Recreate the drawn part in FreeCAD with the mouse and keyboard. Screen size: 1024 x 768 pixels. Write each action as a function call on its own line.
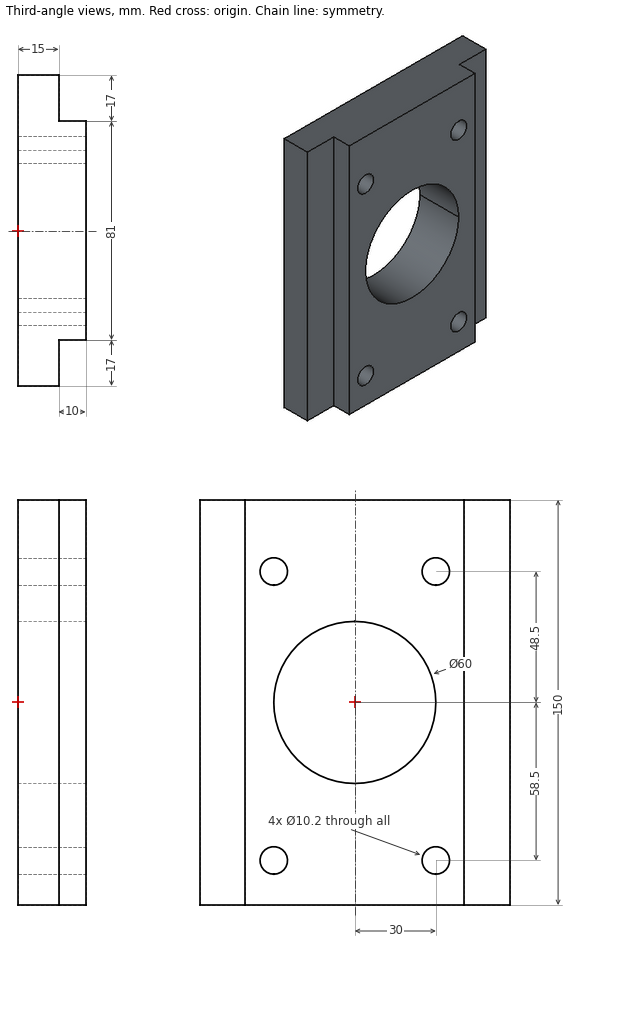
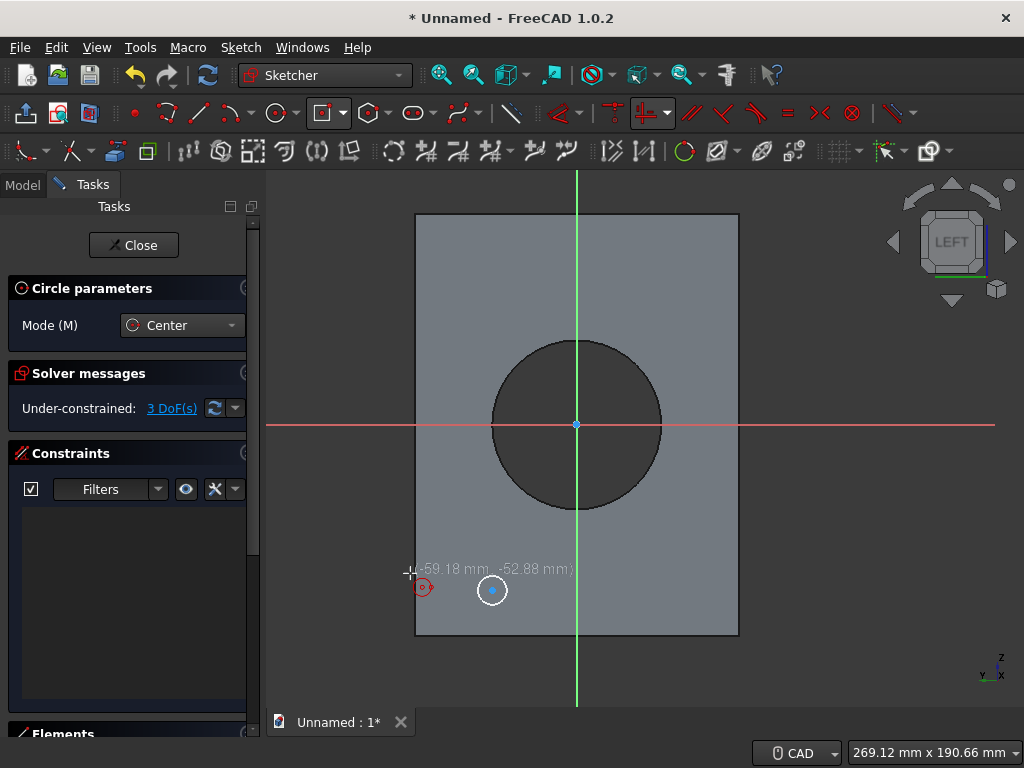
scroll(492, 288, up, 3)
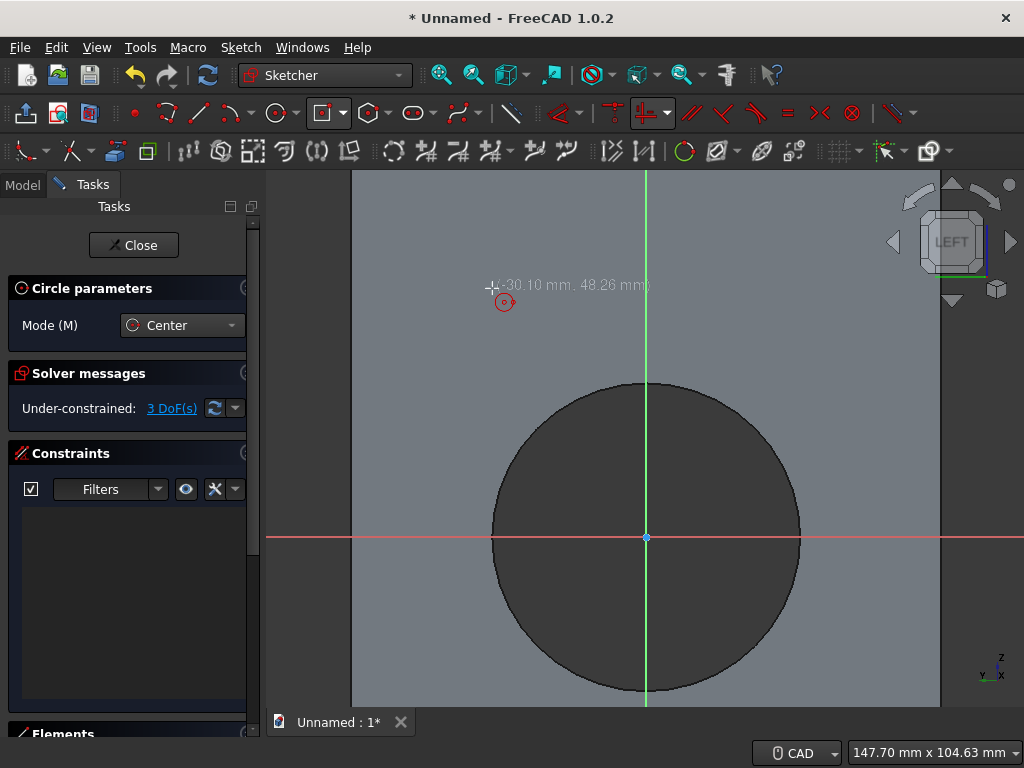
click(492, 288)
click(511, 270)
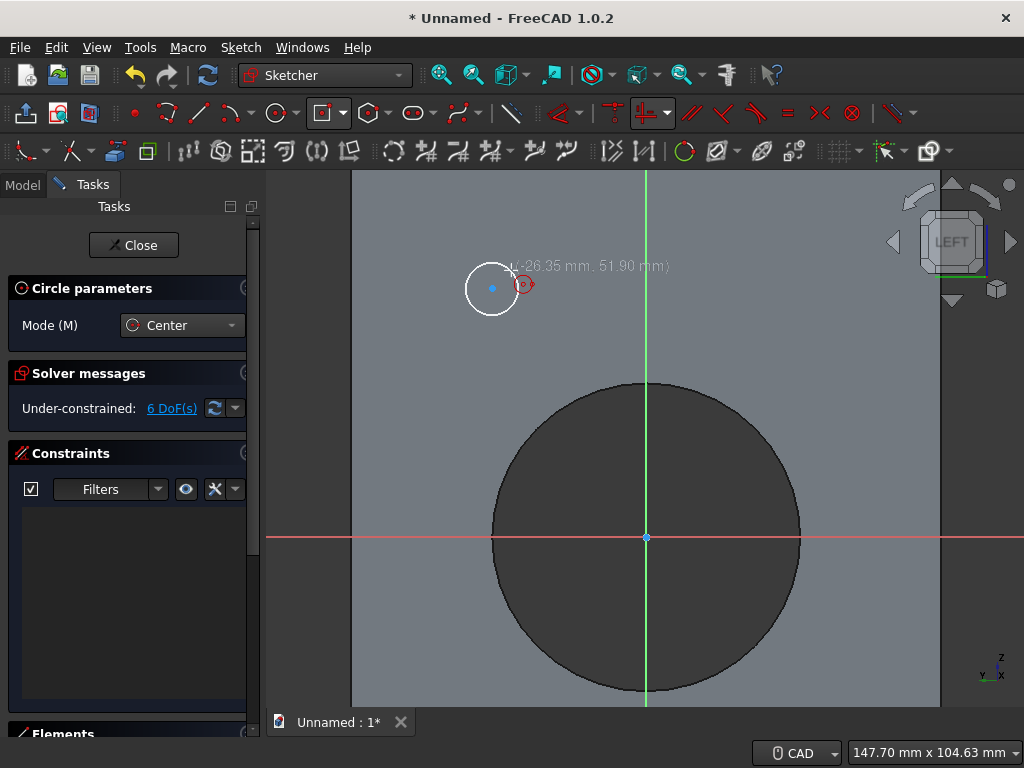
click(800, 288)
click(819, 270)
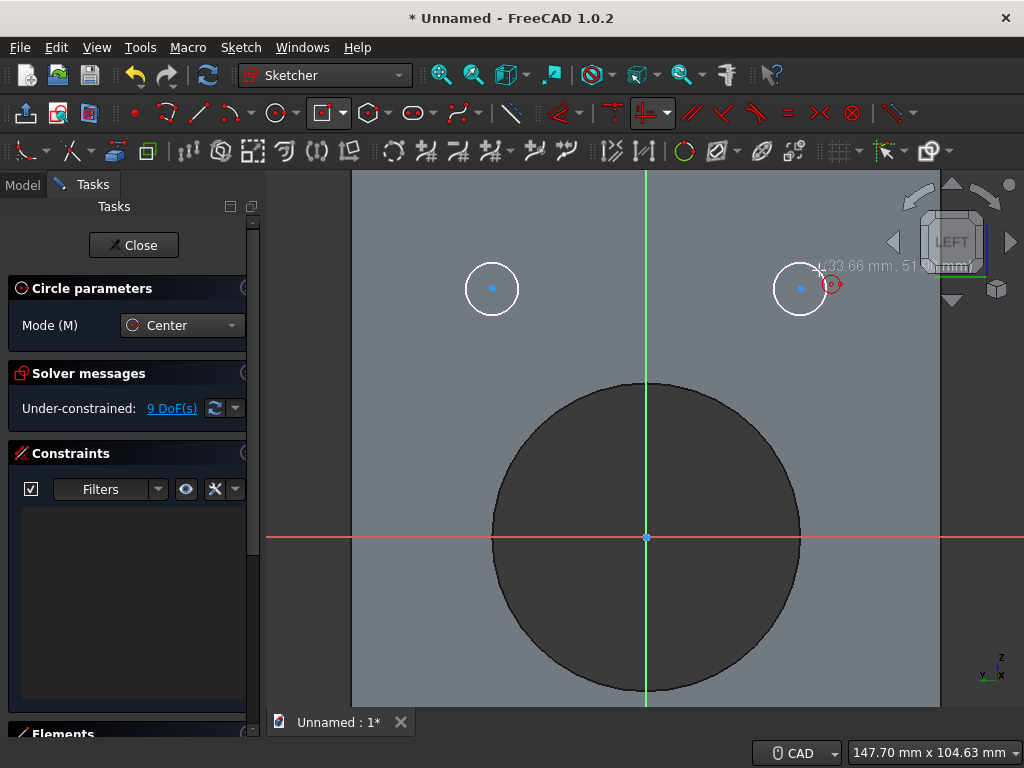
scroll(492, 287, down, 3)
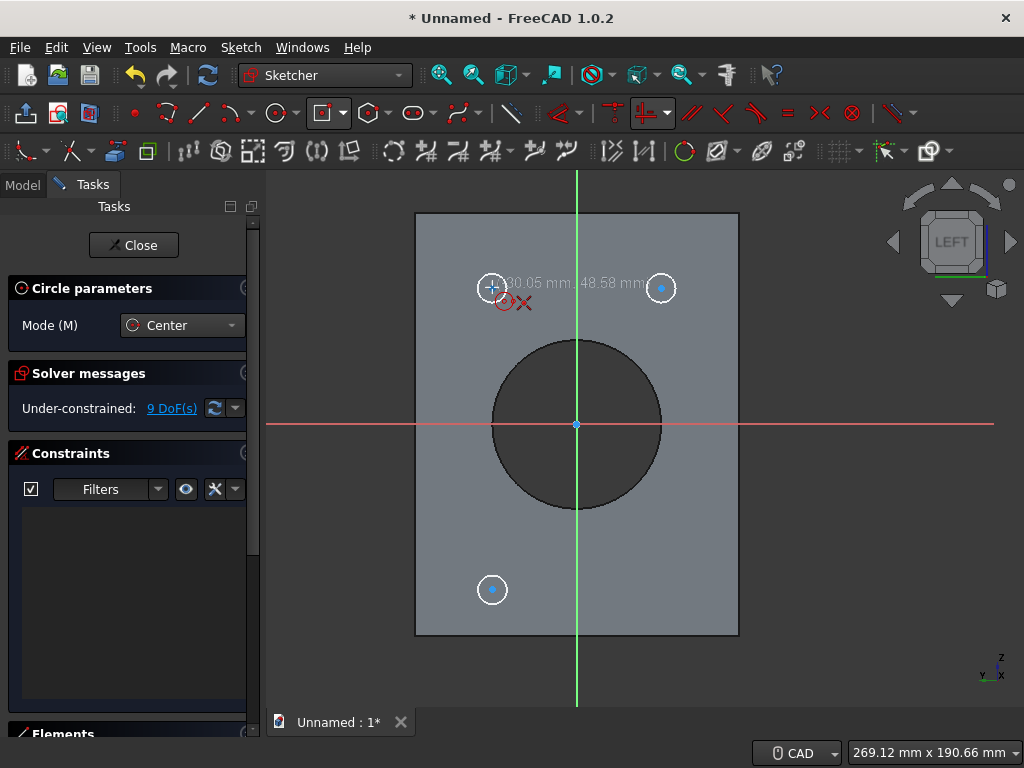
scroll(661, 589, up, 3)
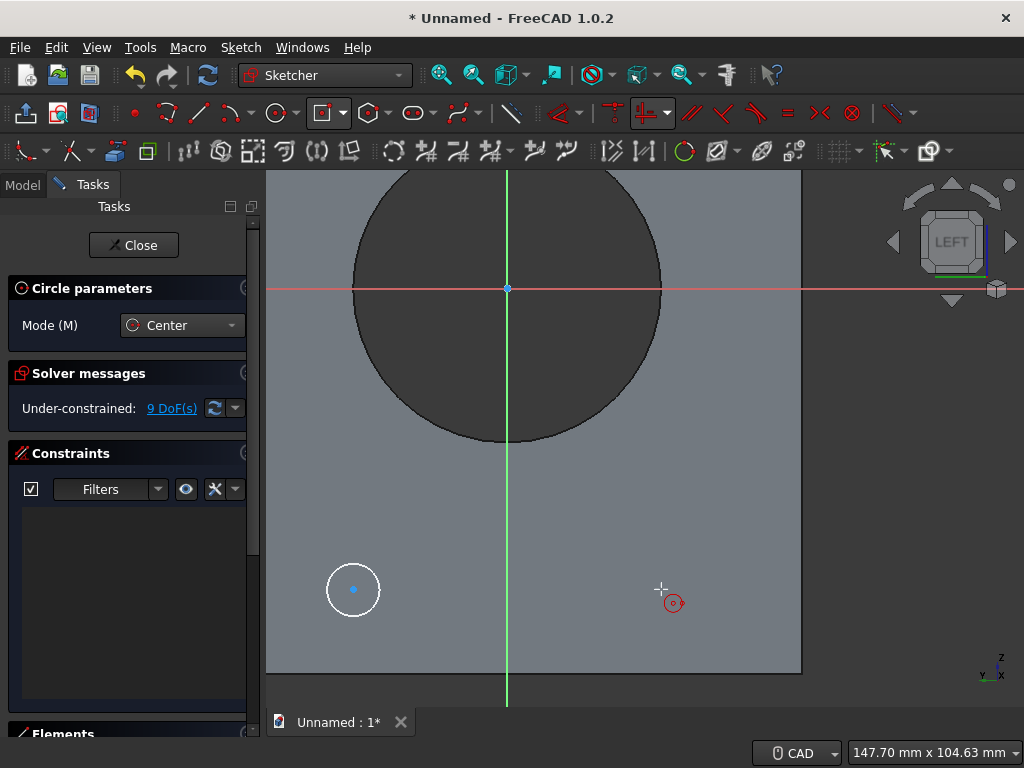
click(661, 589)
click(680, 570)
key(Escape)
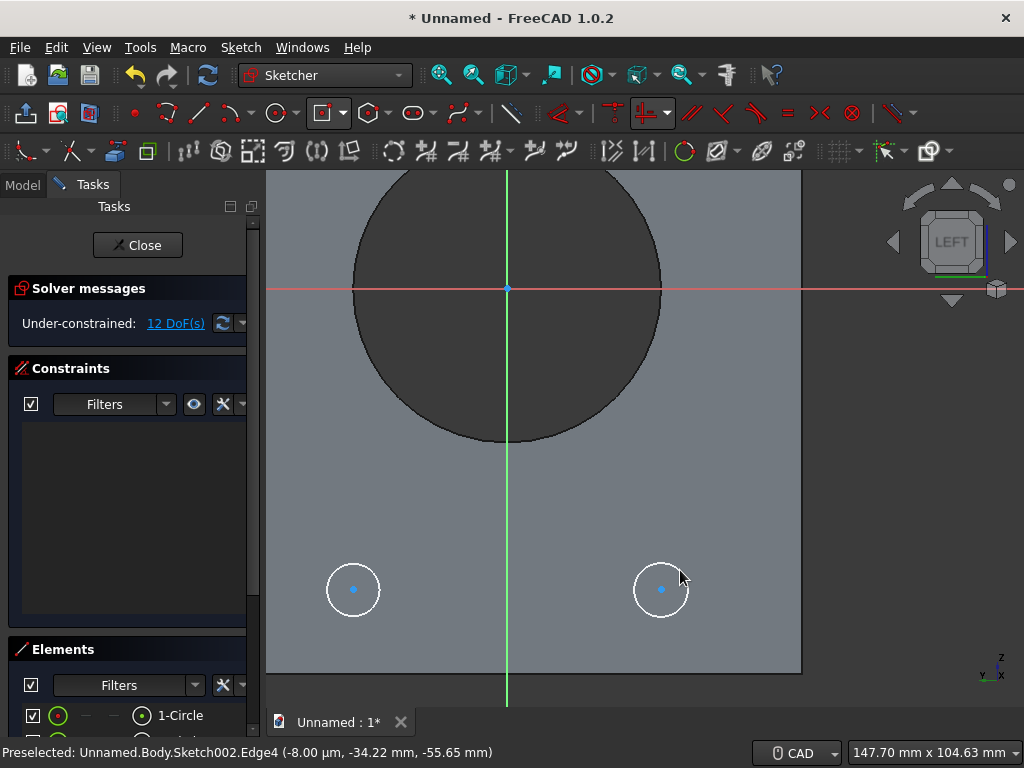
click(372, 571)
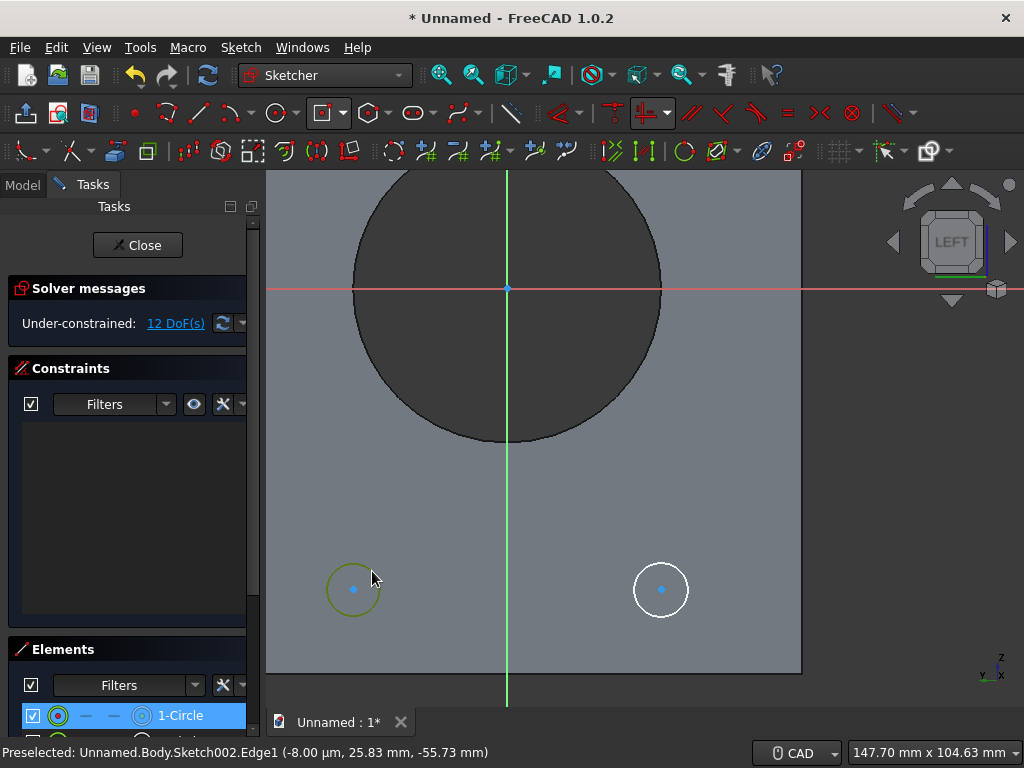
scroll(661, 590, down, 3)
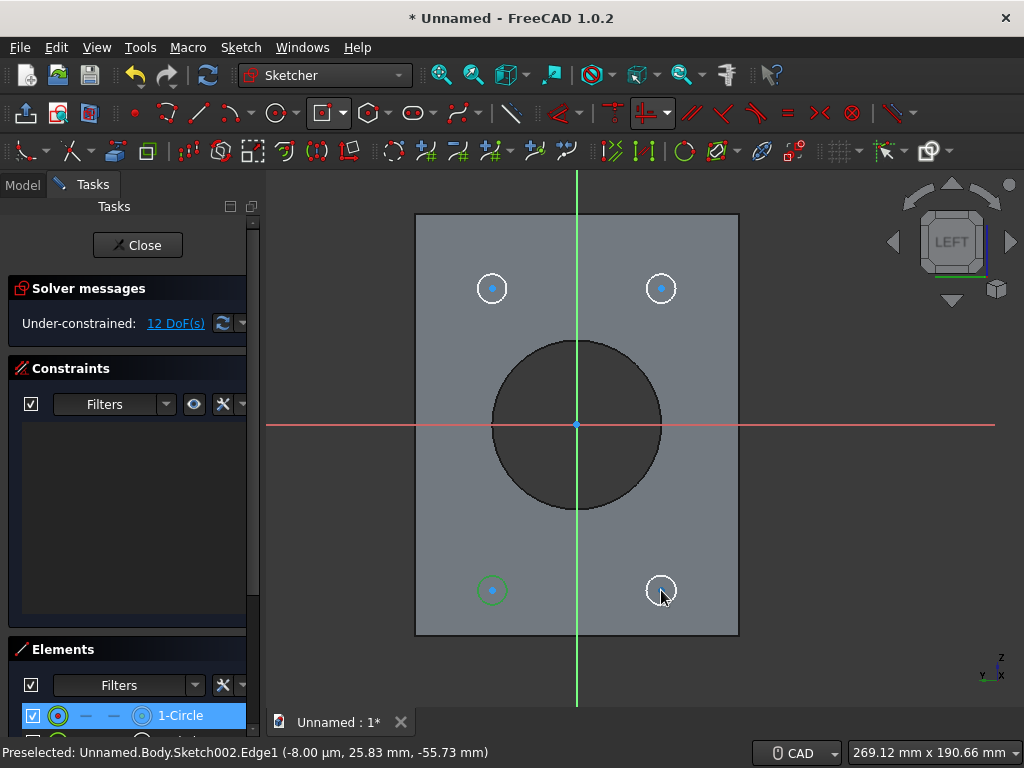
click(502, 278)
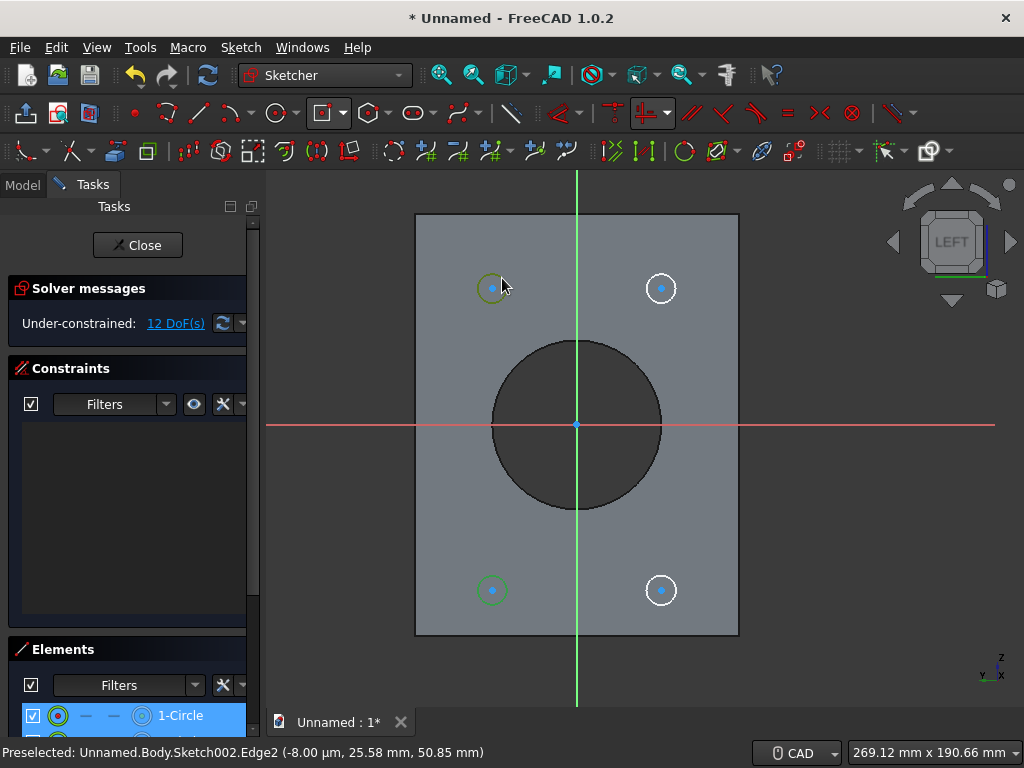
click(671, 278)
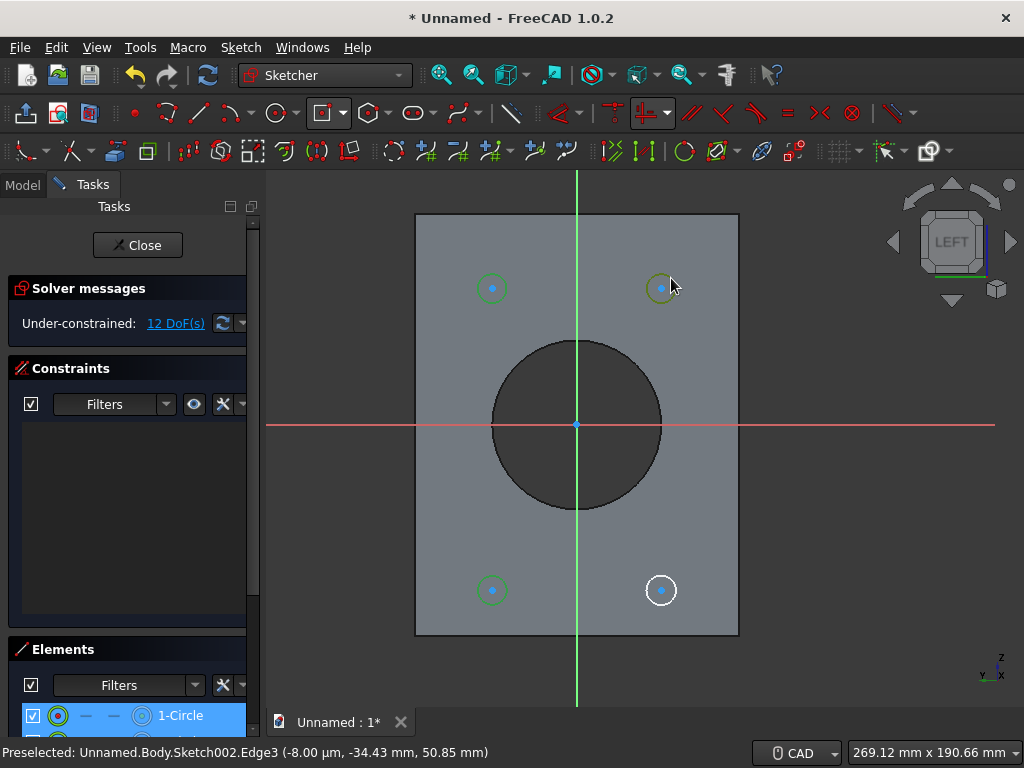
click(672, 580)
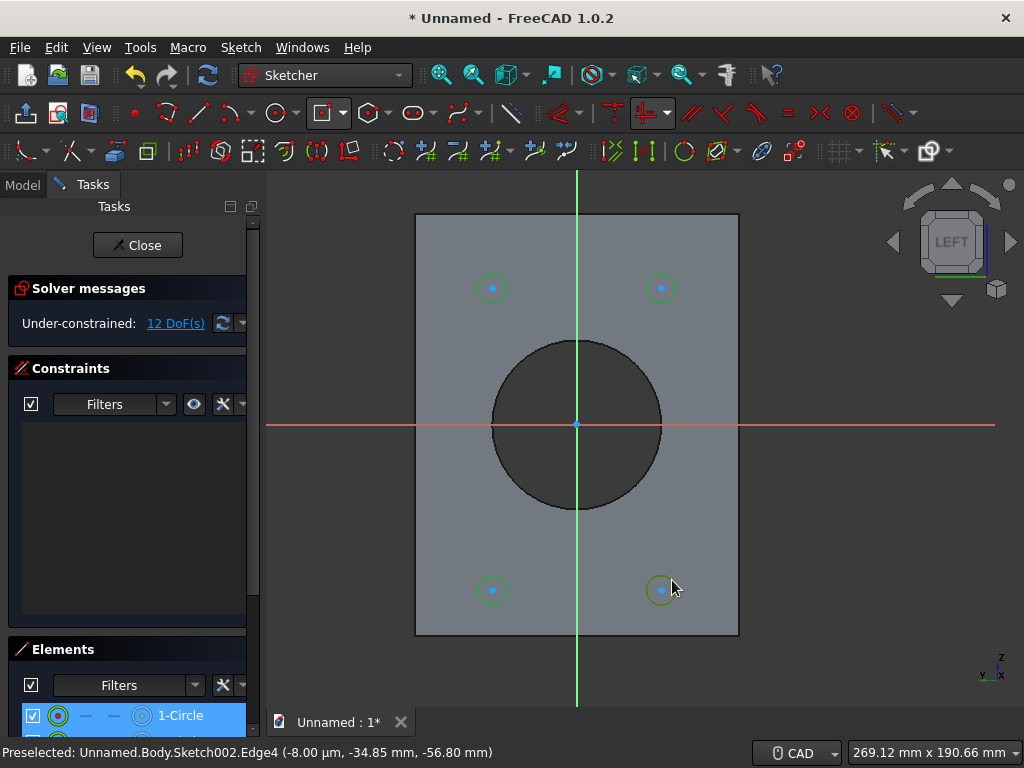
click(788, 114)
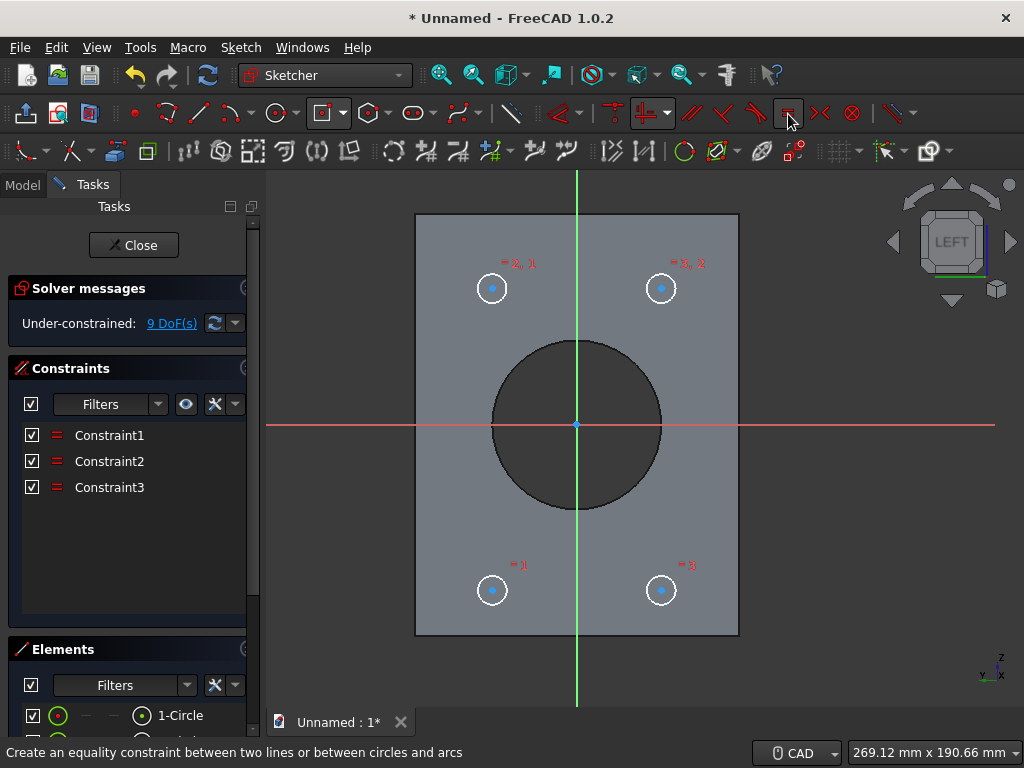
click(492, 289)